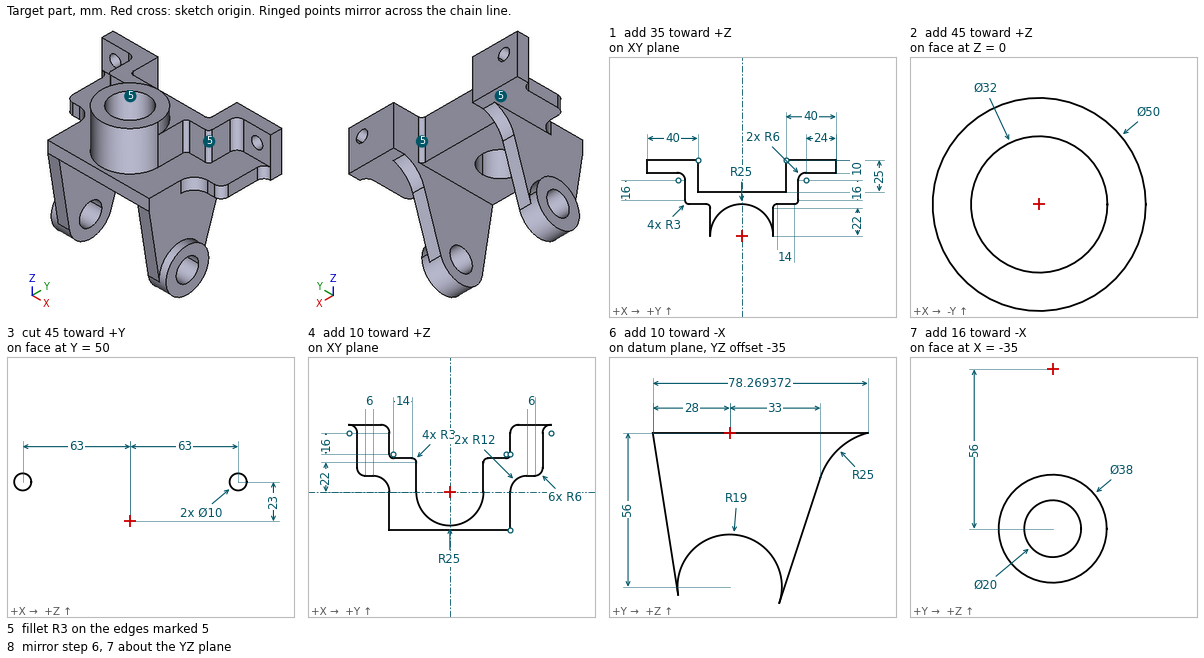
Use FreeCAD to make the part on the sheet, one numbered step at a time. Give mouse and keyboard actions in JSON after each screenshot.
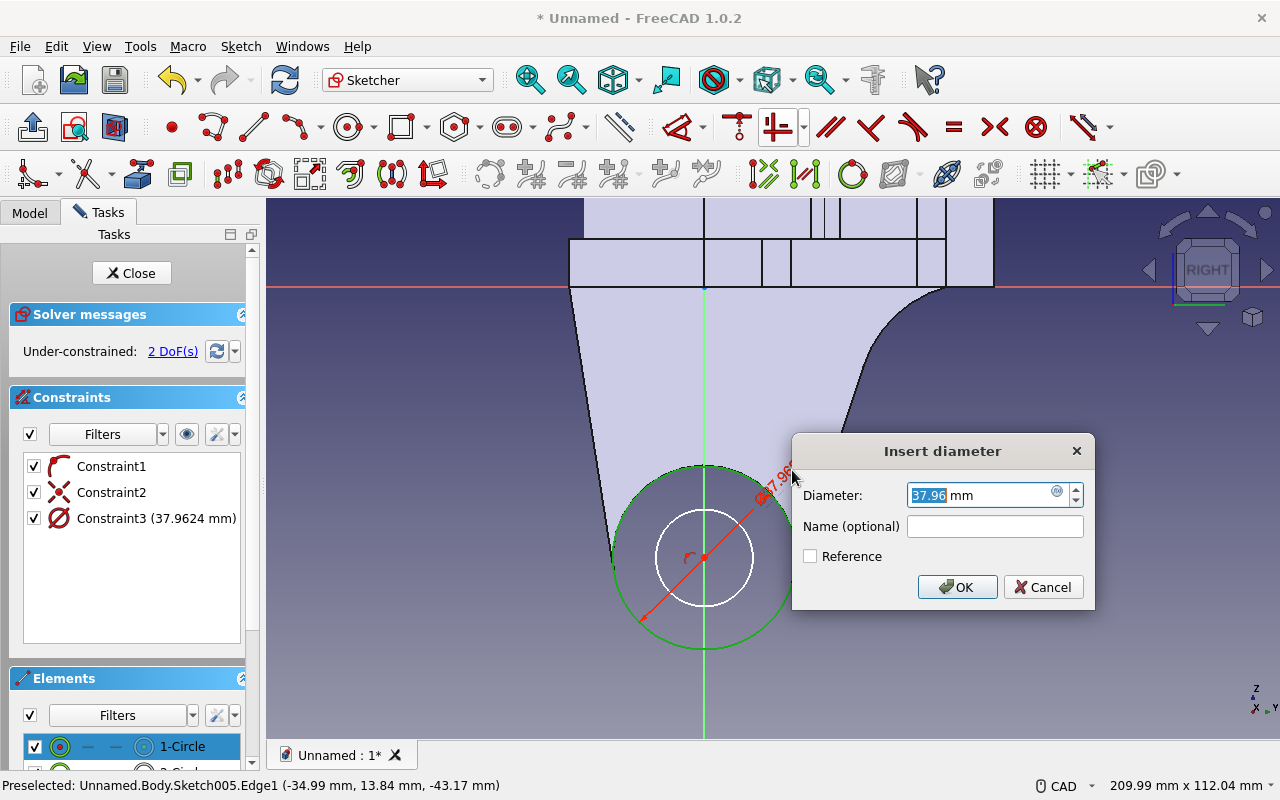
{"action": "type", "text": "38"}
{"action": "key", "text": "Return"}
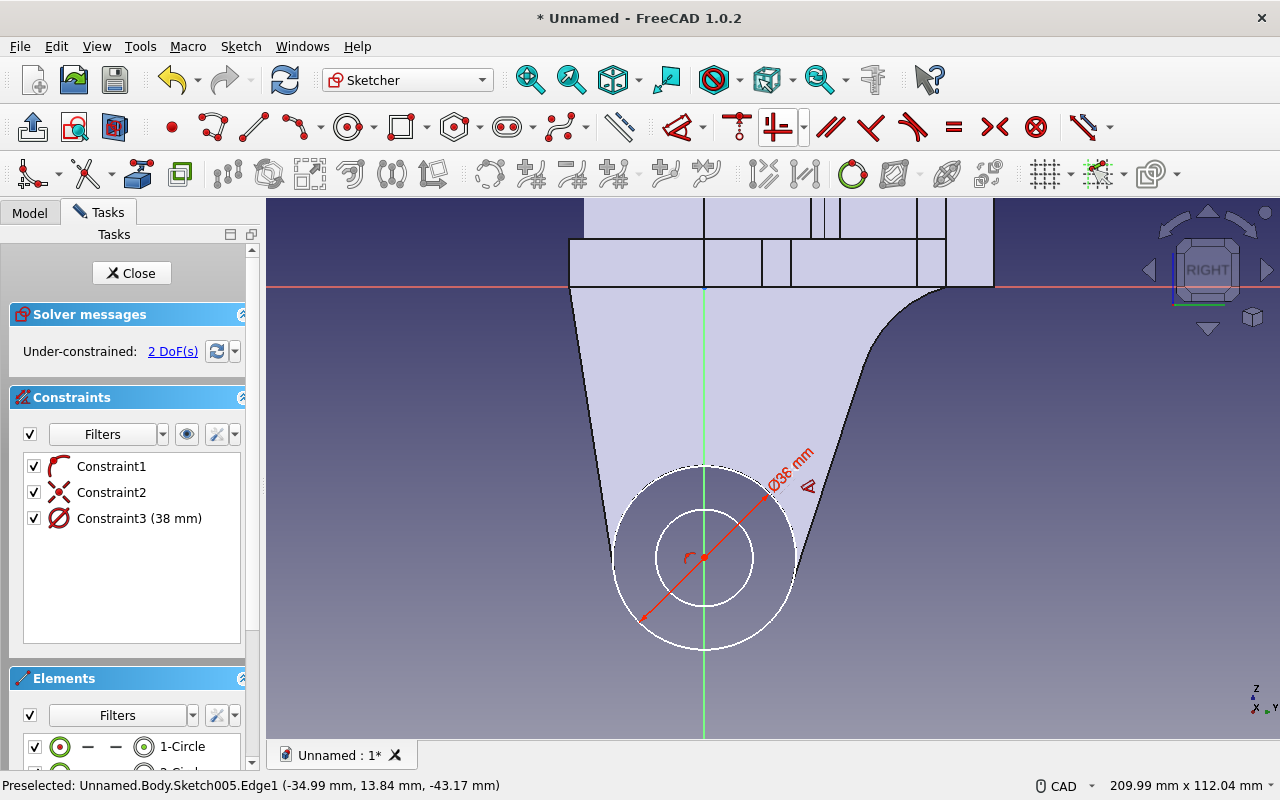
{"action": "left_click", "coordinate": [739, 524]}
{"action": "left_click", "coordinate": [828, 523]}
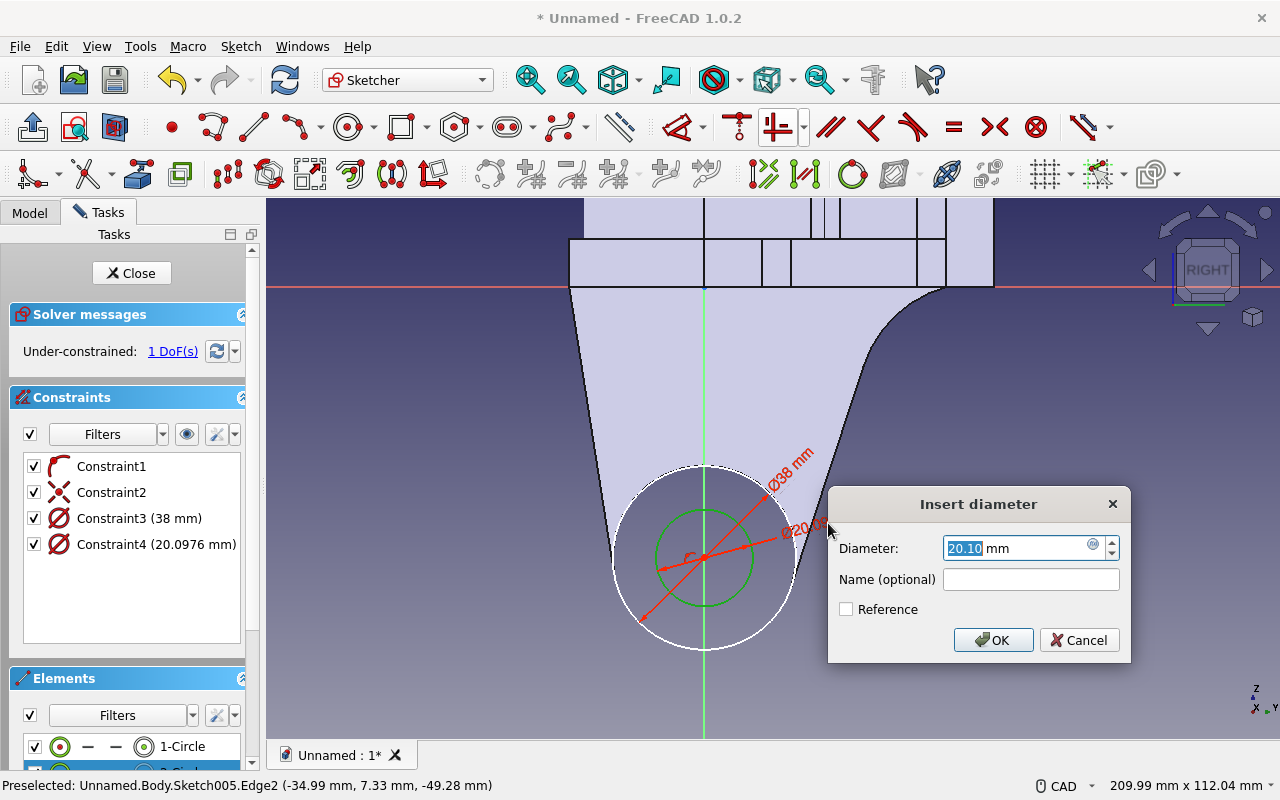
{"action": "type", "text": "20"}
{"action": "key", "text": "Return"}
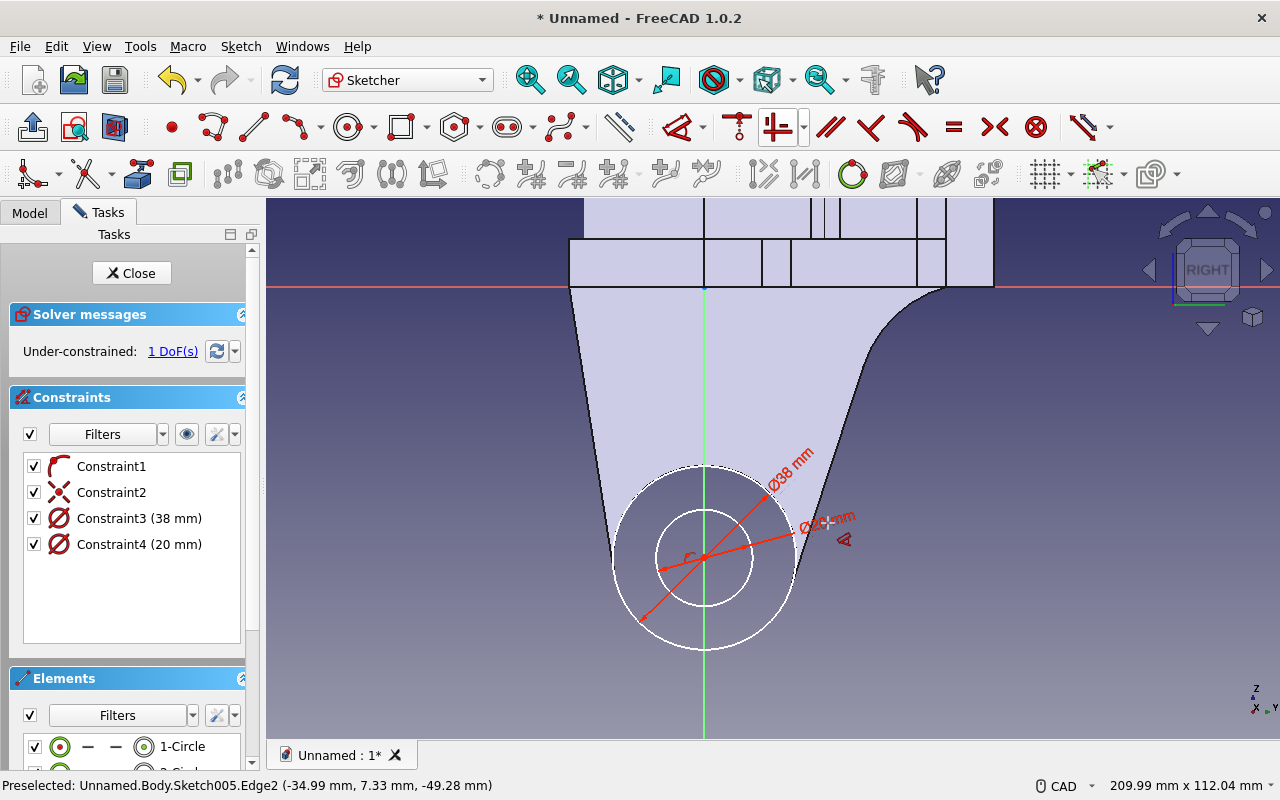
{"action": "left_click", "coordinate": [704, 558]}
{"action": "left_click", "coordinate": [738, 422]}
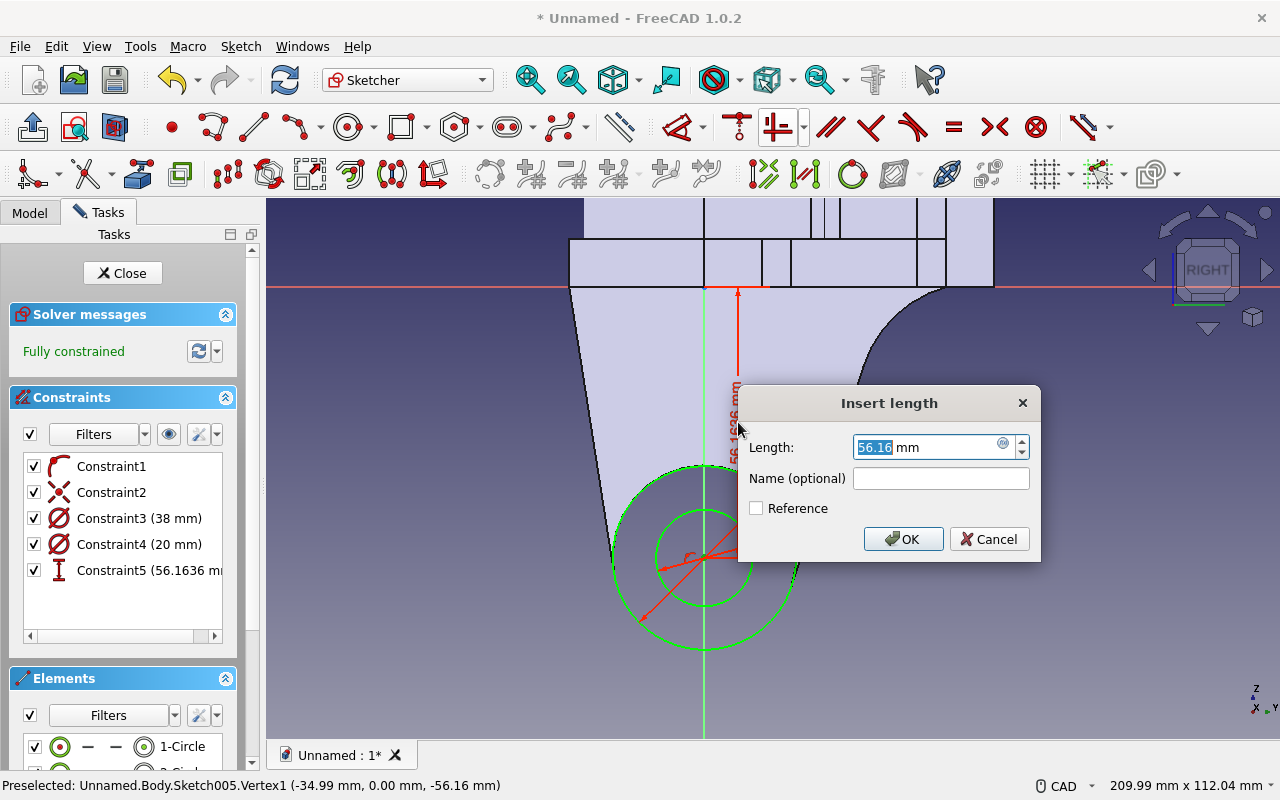
{"action": "type", "text": "56"}
{"action": "key", "text": "Return"}
{"action": "key", "text": "Escape"}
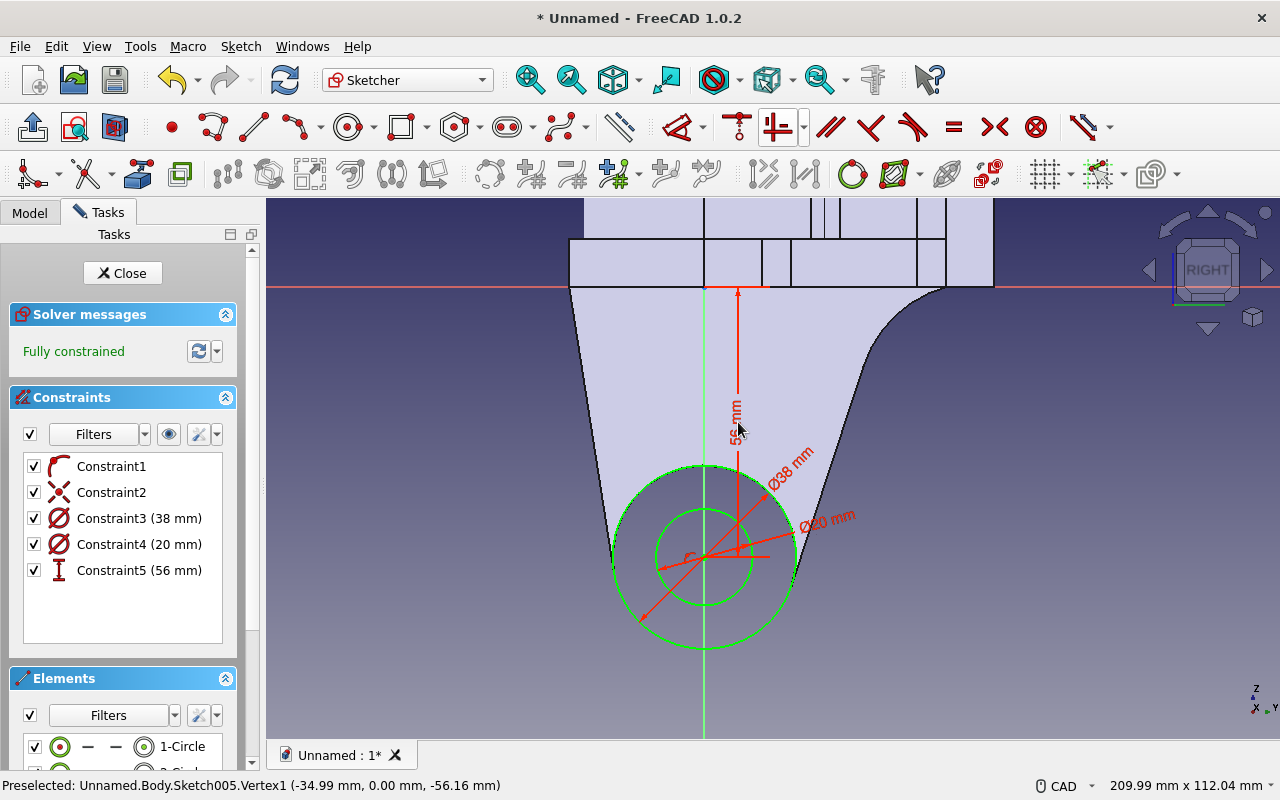
{"action": "left_click", "coordinate": [123, 273]}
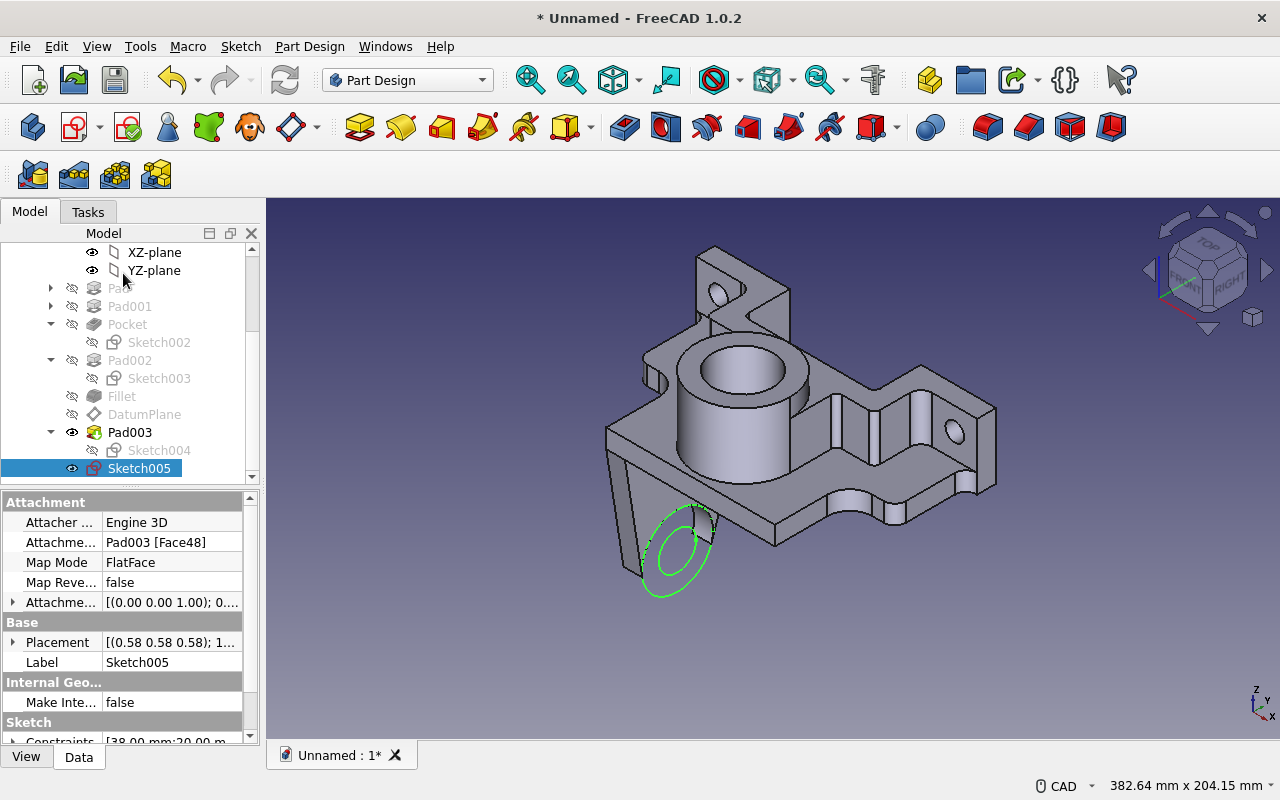
{"action": "left_click", "coordinate": [360, 128]}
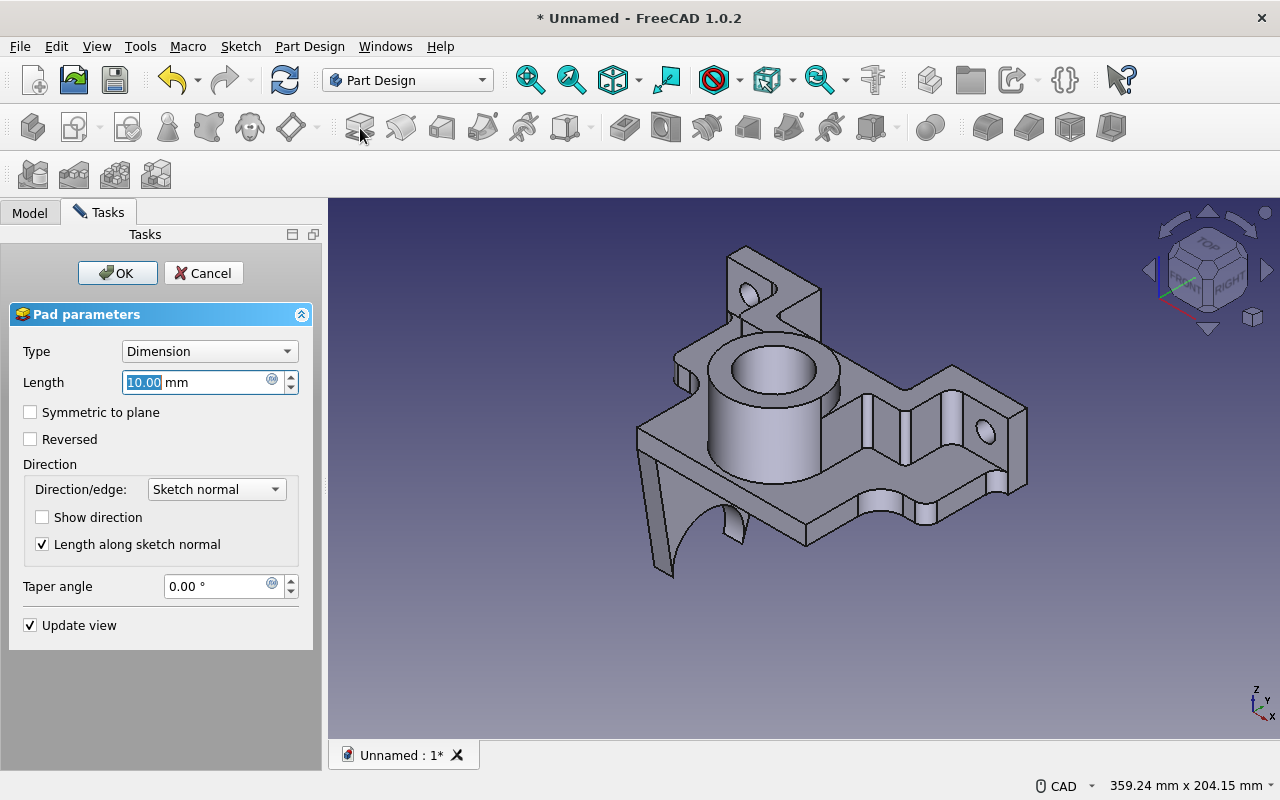
{"action": "type", "text": "16"}
{"action": "key", "text": "Tab"}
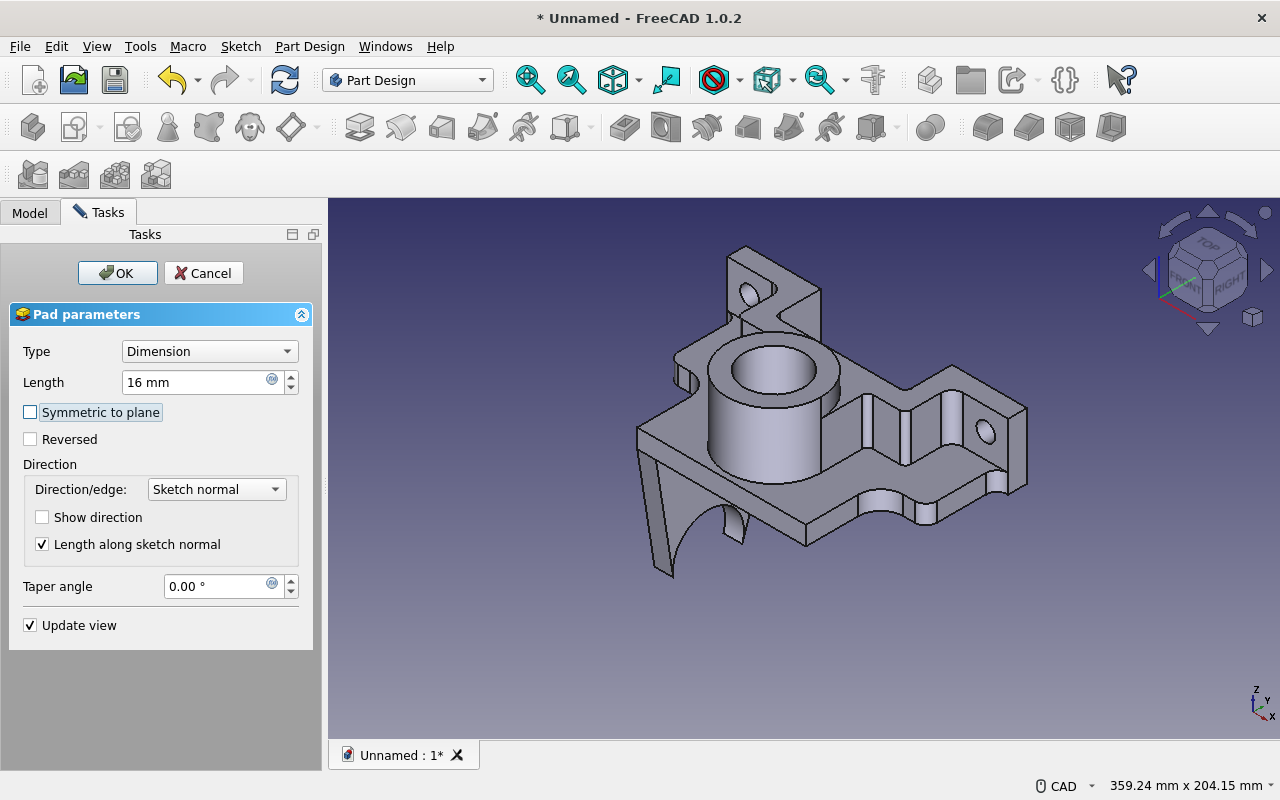
{"action": "left_click", "coordinate": [31, 439]}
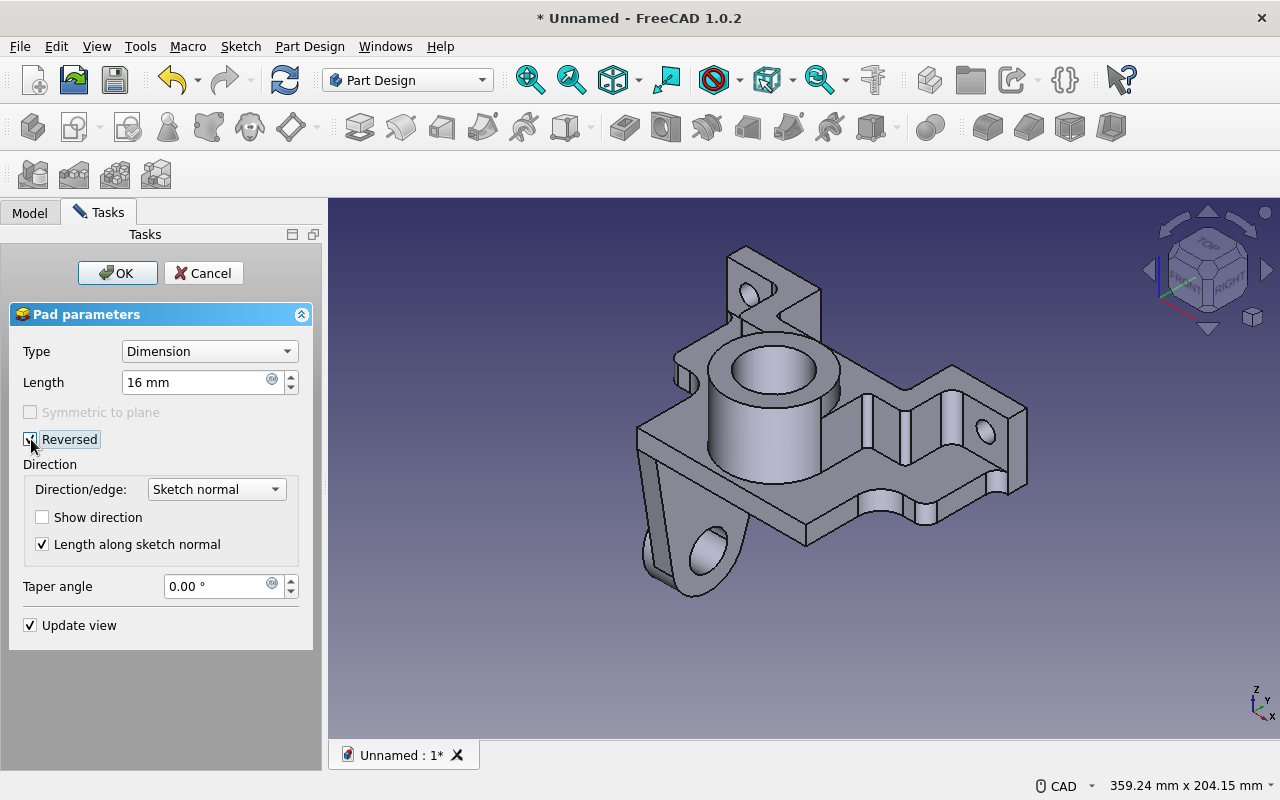
{"action": "left_click", "coordinate": [118, 273]}